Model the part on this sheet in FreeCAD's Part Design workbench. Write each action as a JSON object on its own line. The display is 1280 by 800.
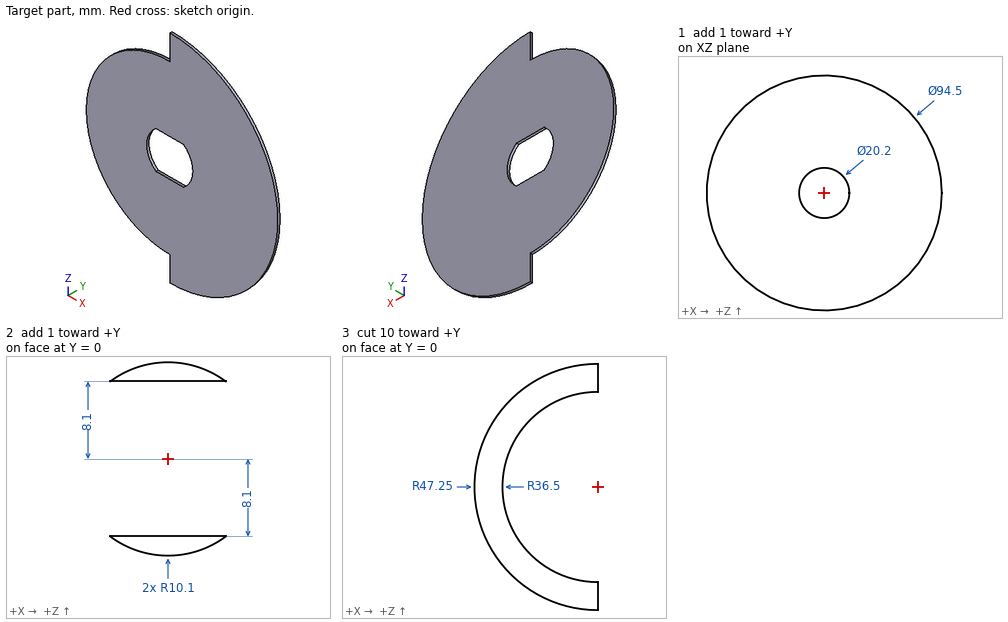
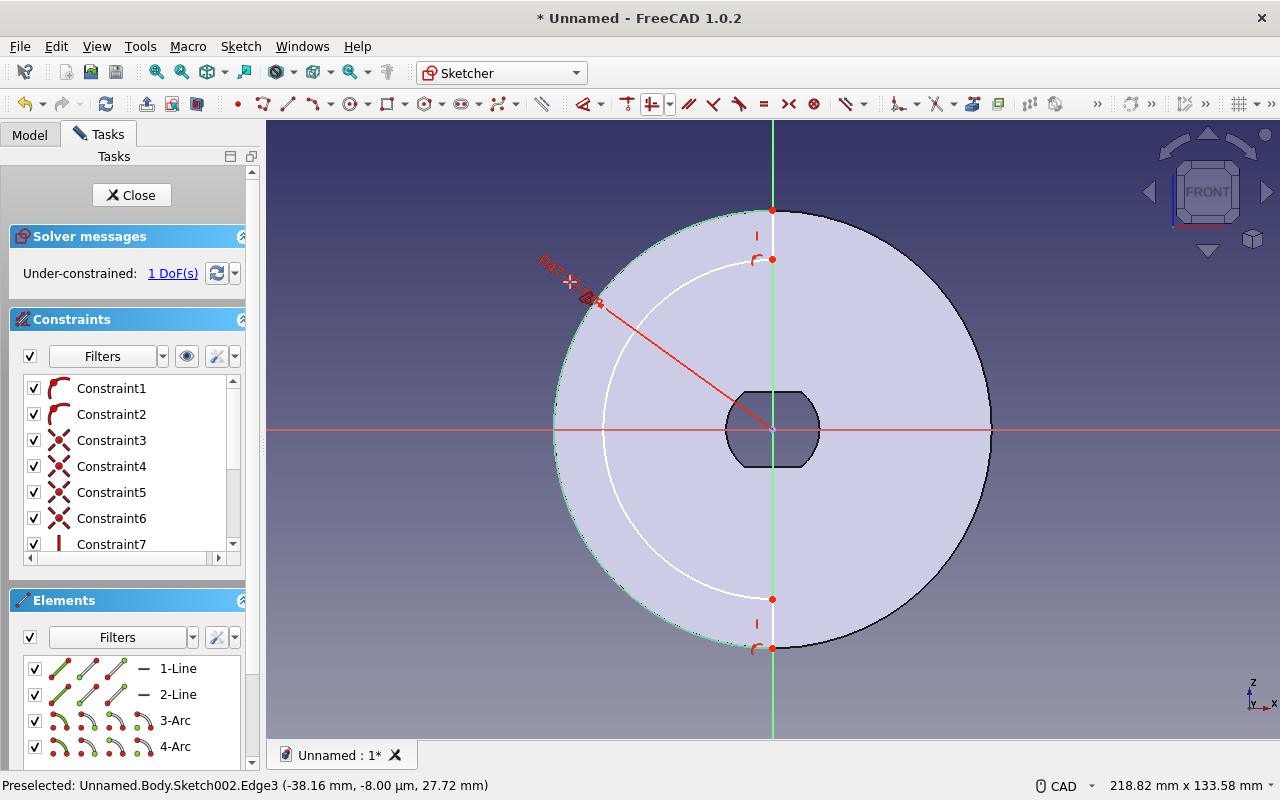
{"action": "left_click", "coordinate": [636, 330]}
{"action": "left_click", "coordinate": [610, 311]}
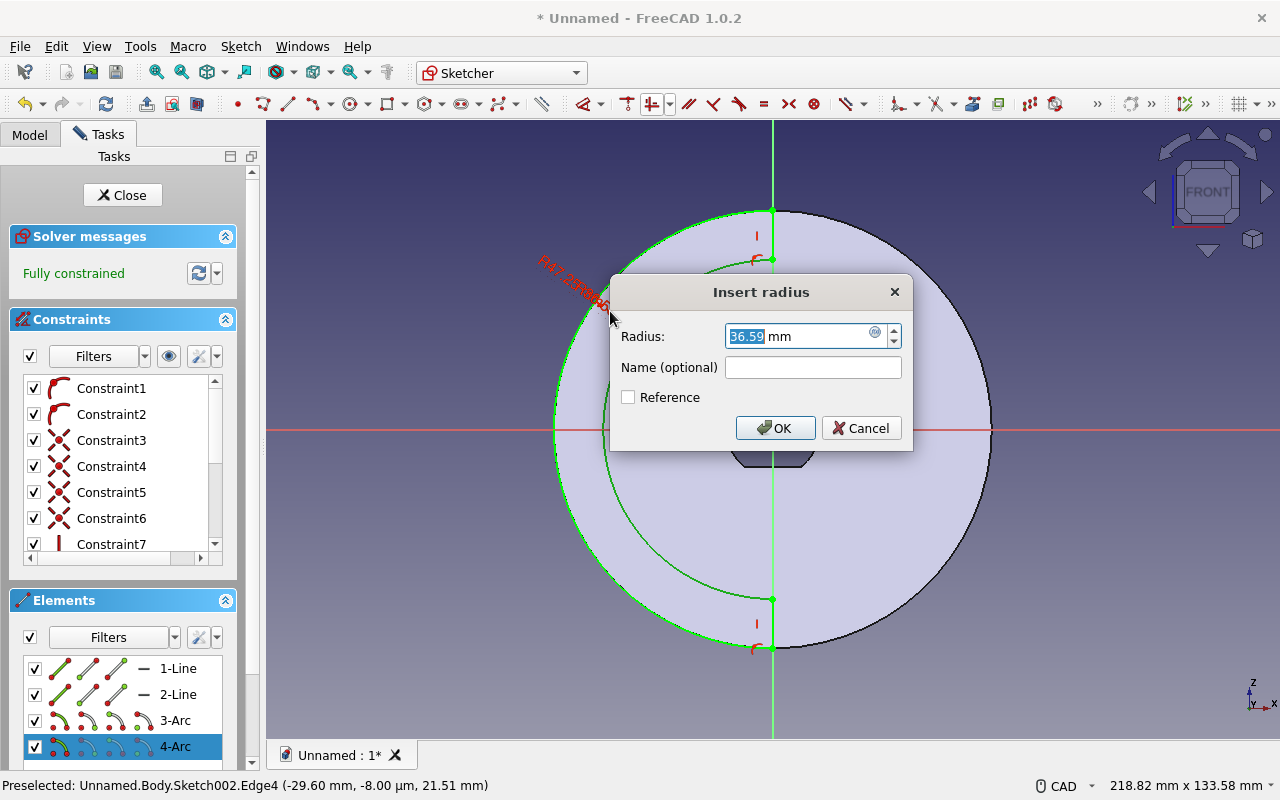
{"action": "type", "text": "36.5"}
{"action": "key", "text": "Return"}
{"action": "key", "text": "Escape"}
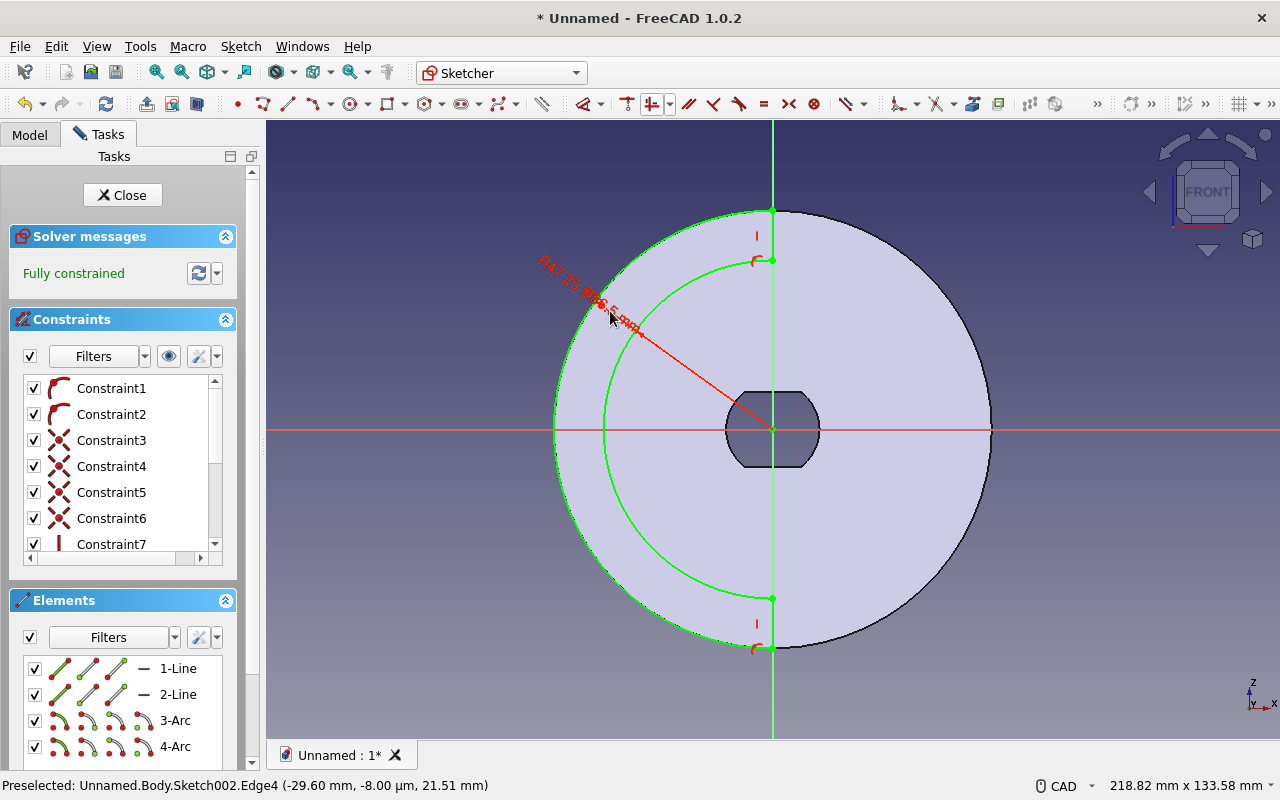
{"action": "left_click", "coordinate": [123, 195]}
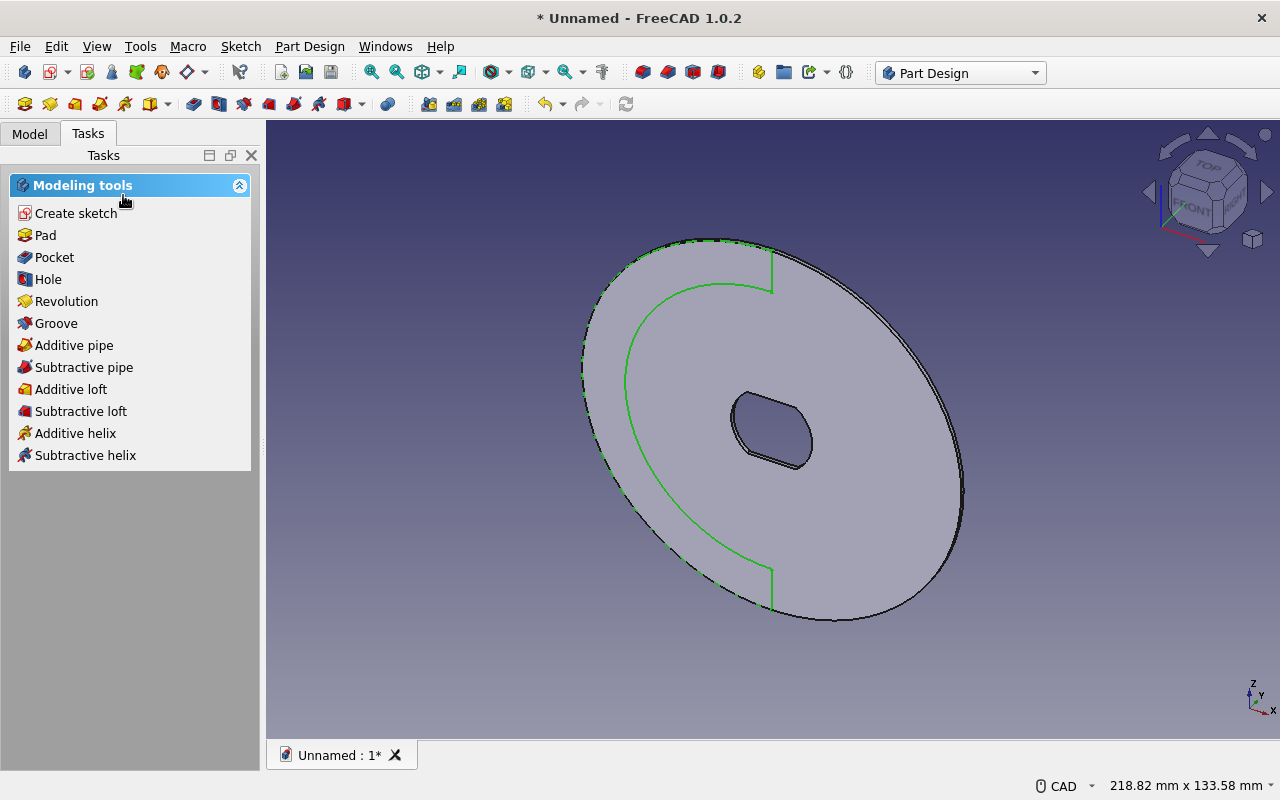
{"action": "left_click", "coordinate": [194, 104]}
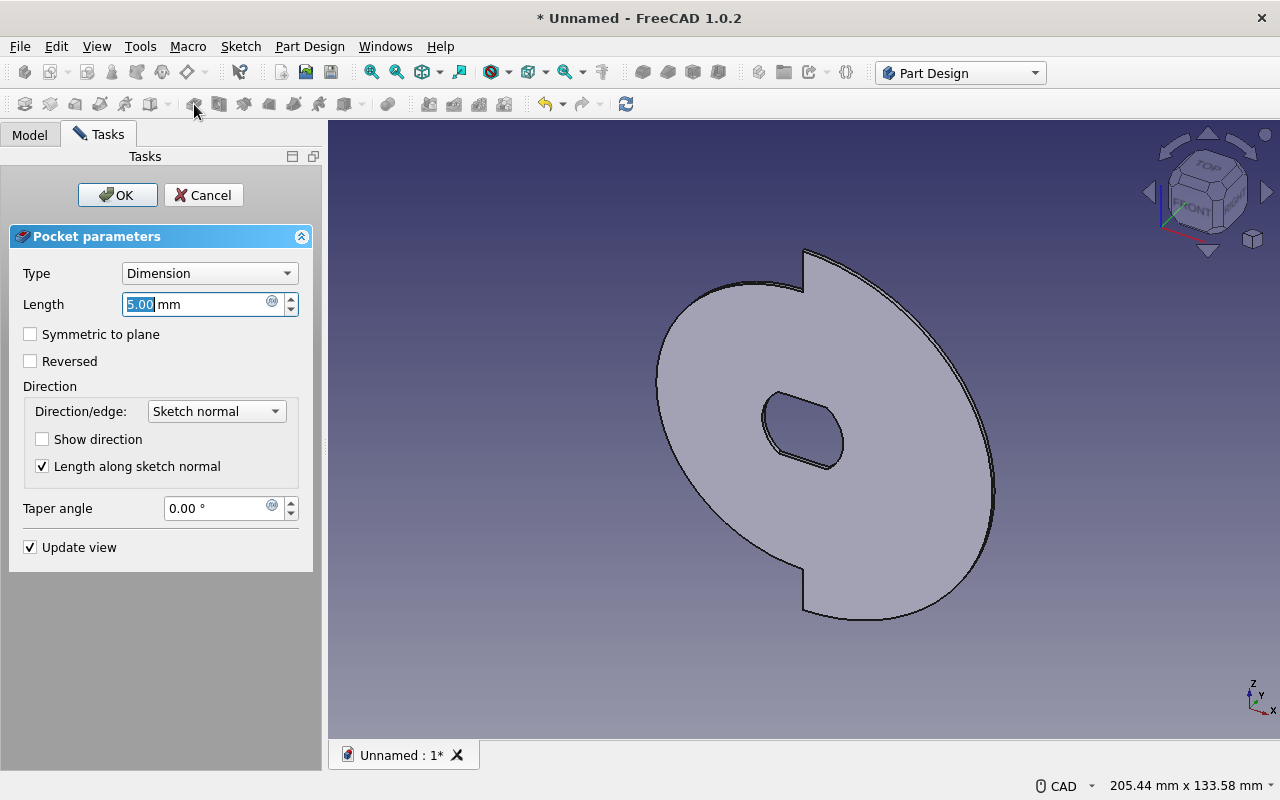
{"action": "type", "text": "10"}
{"action": "key", "text": "Tab"}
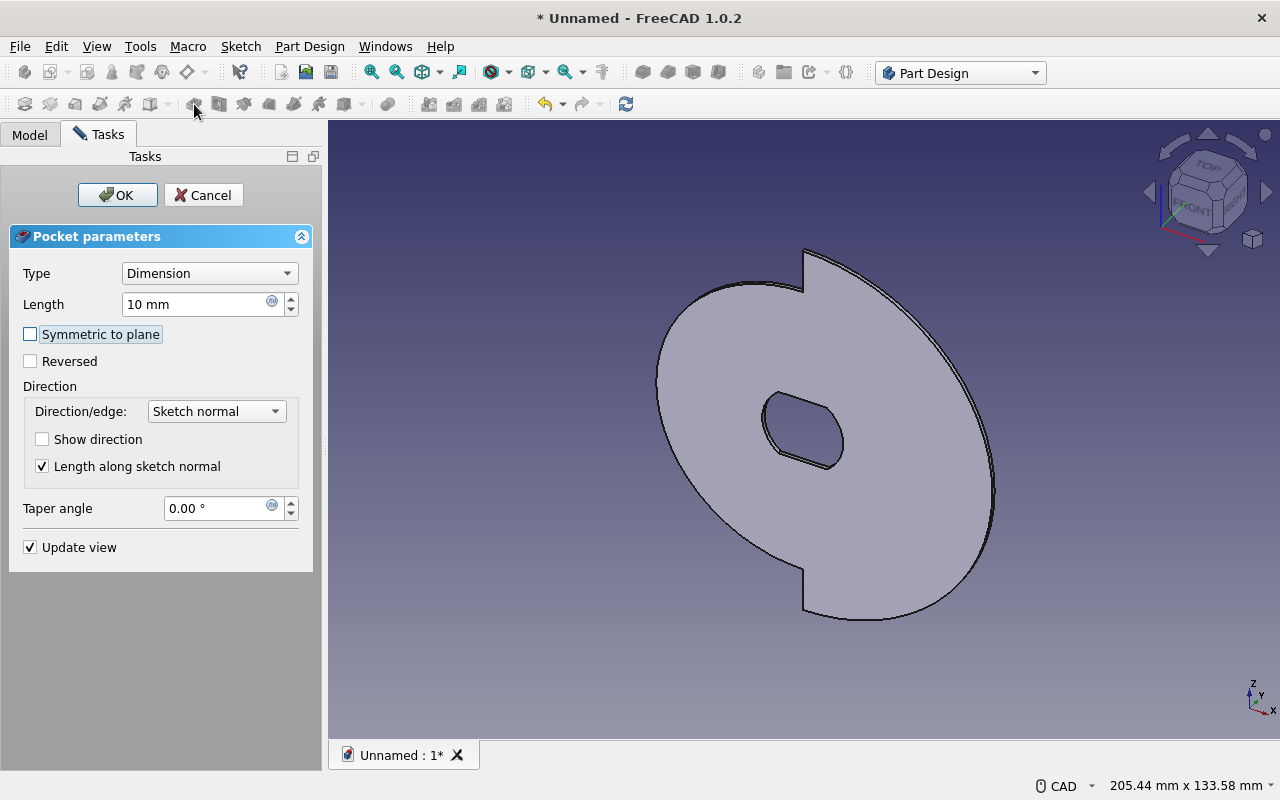
{"action": "left_click", "coordinate": [118, 195]}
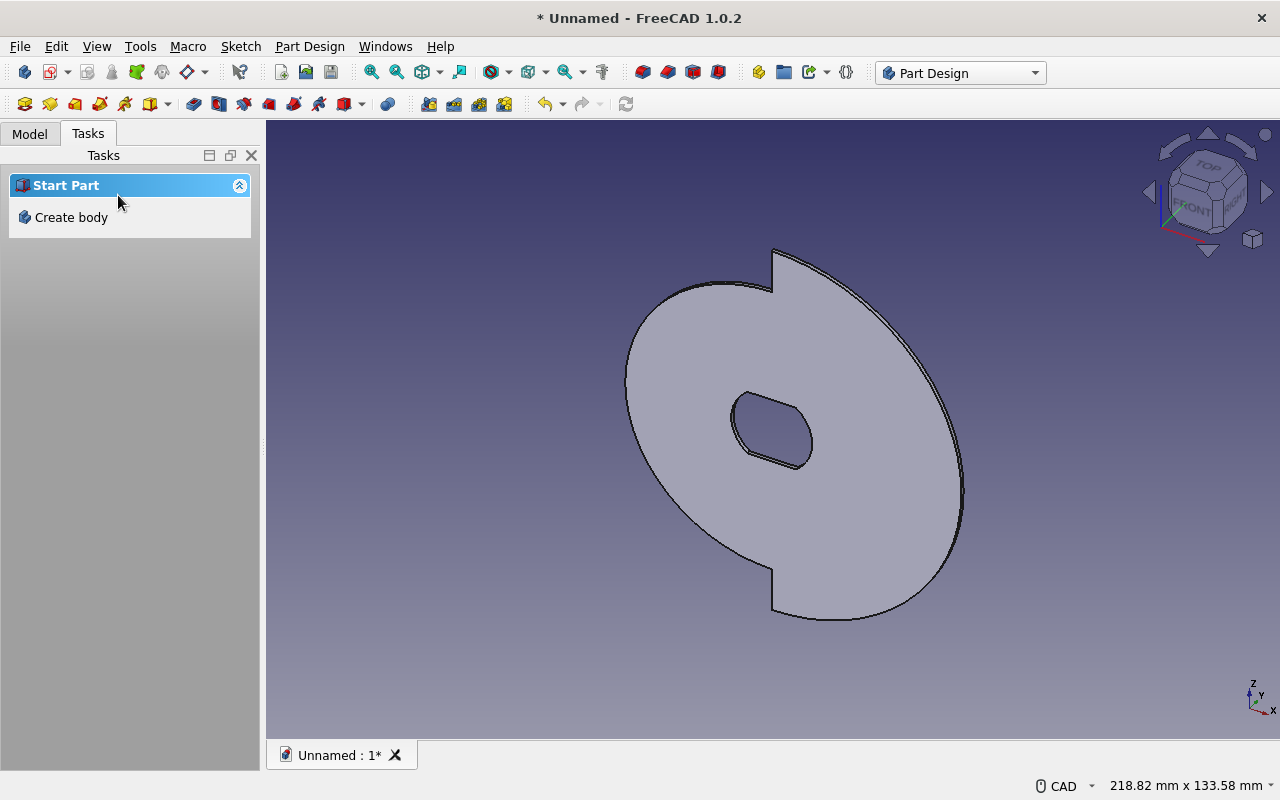
{"action": "key", "text": "0"}